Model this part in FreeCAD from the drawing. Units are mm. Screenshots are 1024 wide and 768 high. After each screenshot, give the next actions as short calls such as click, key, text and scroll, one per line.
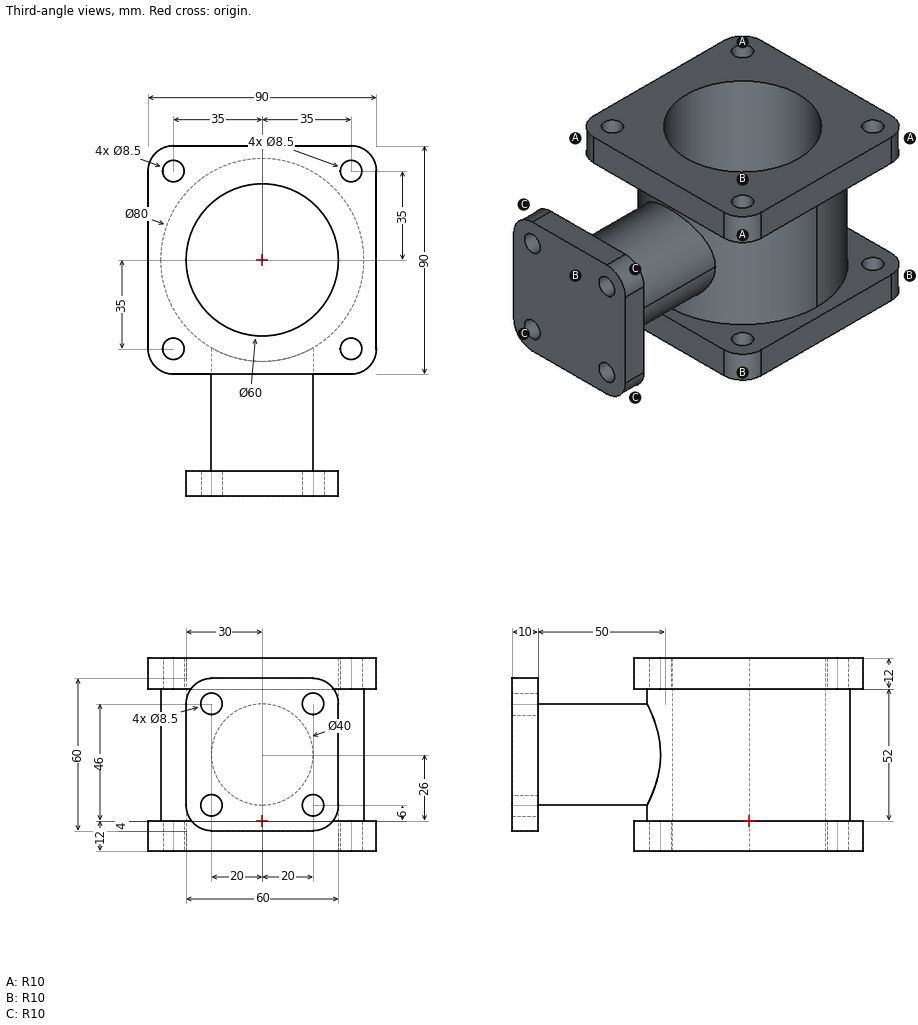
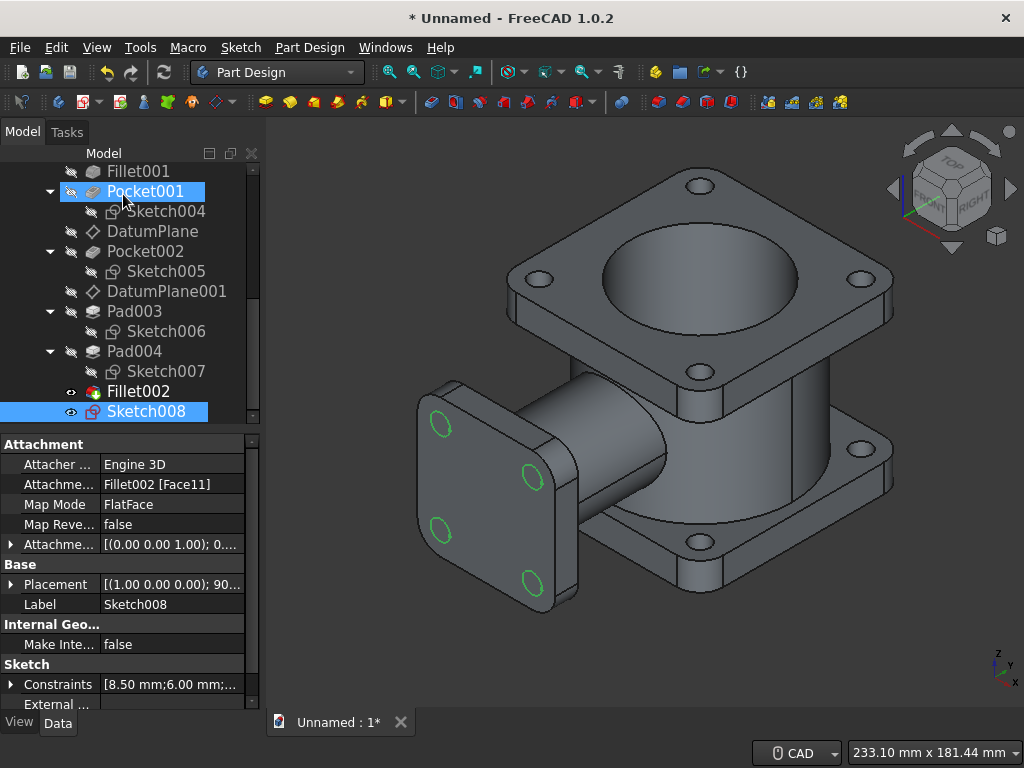
click(432, 102)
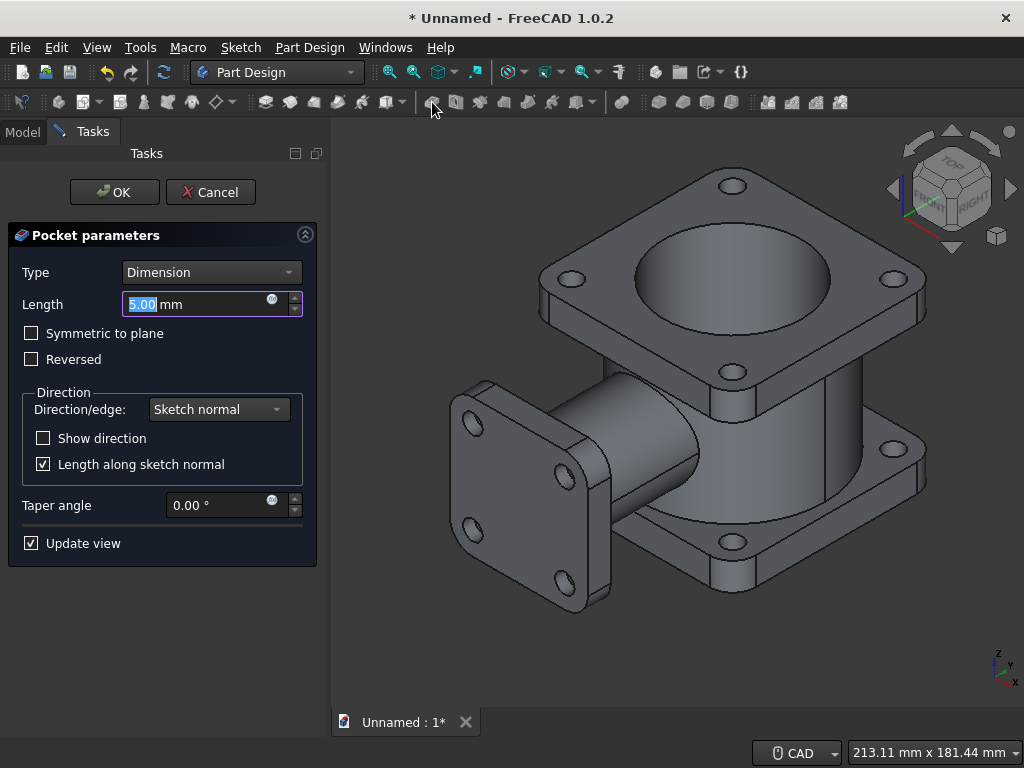
text(10)
key(Tab)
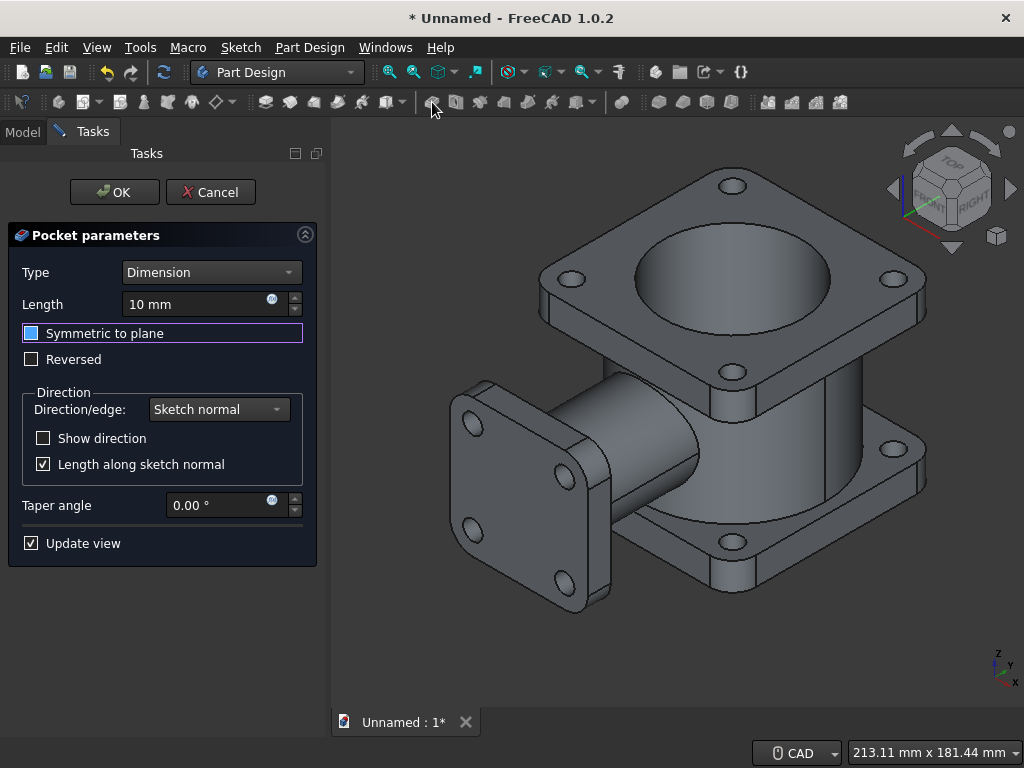
click(115, 192)